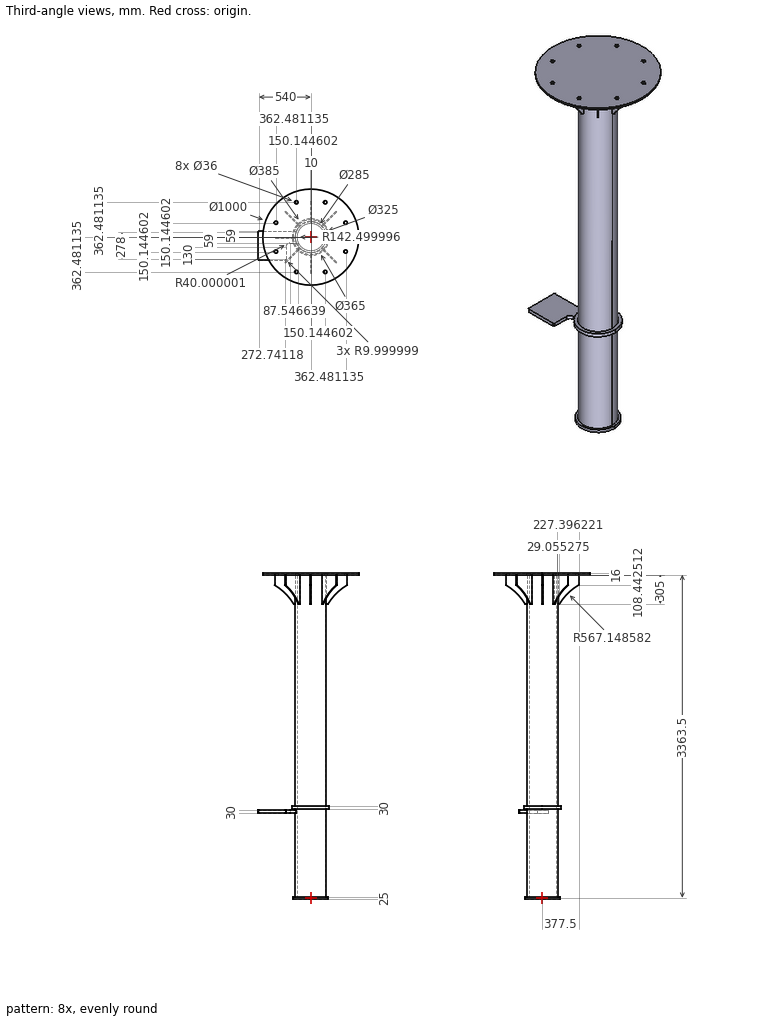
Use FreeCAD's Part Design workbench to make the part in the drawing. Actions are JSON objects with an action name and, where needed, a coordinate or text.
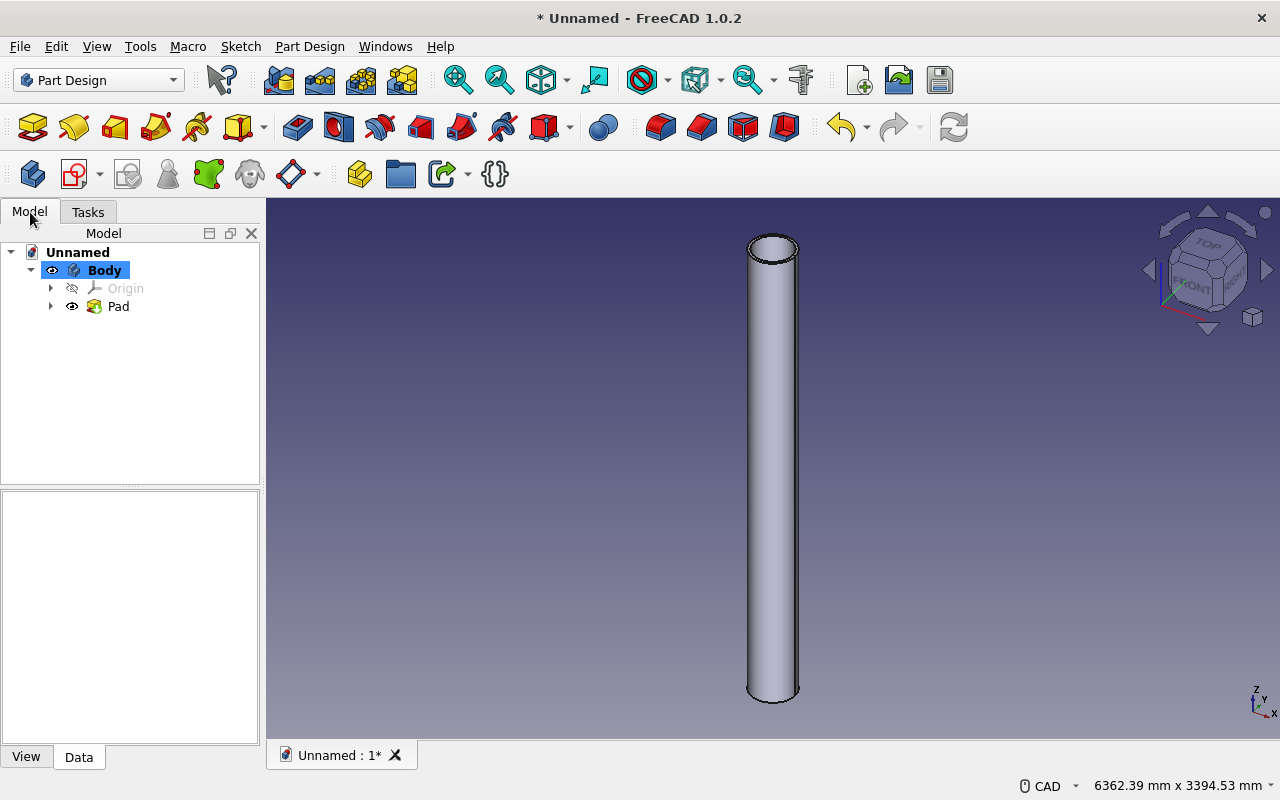
{"action": "left_click", "coordinate": [51, 288]}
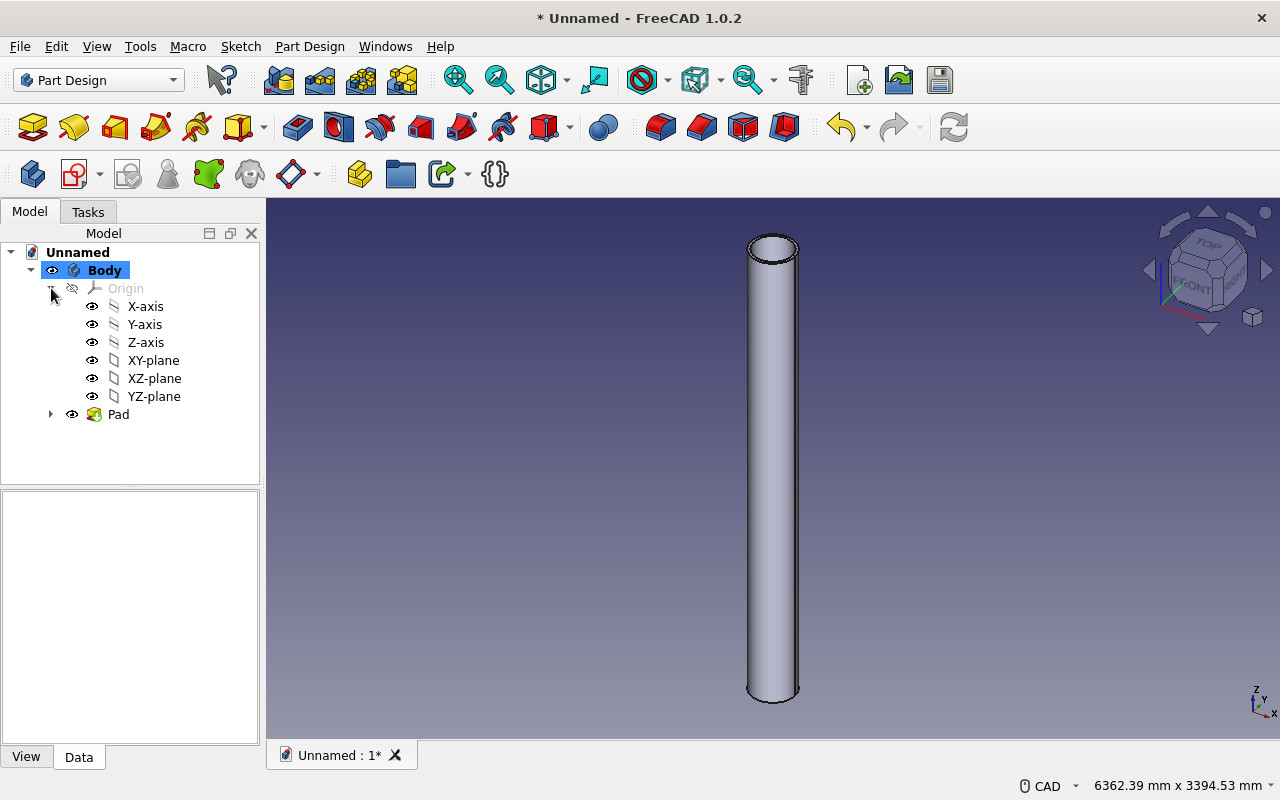
{"action": "left_click", "coordinate": [137, 360]}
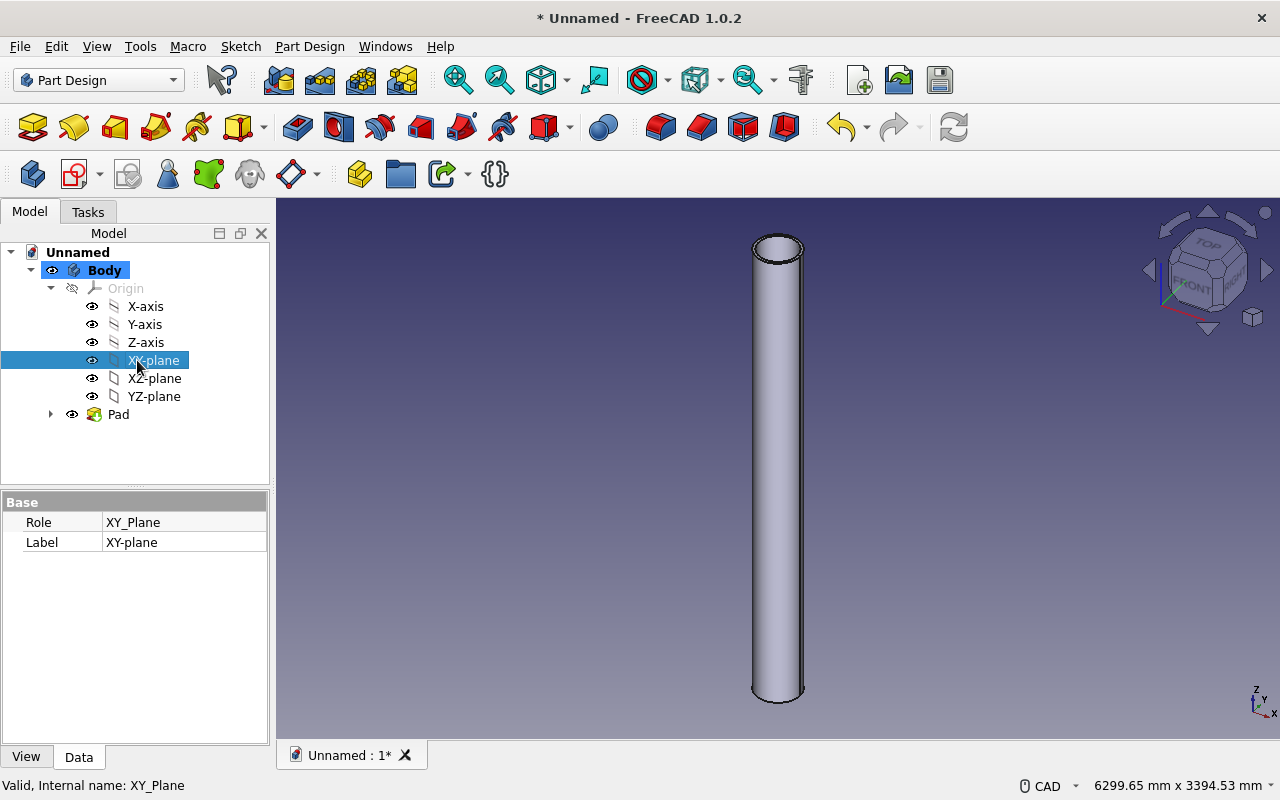
{"action": "left_click", "coordinate": [290, 174]}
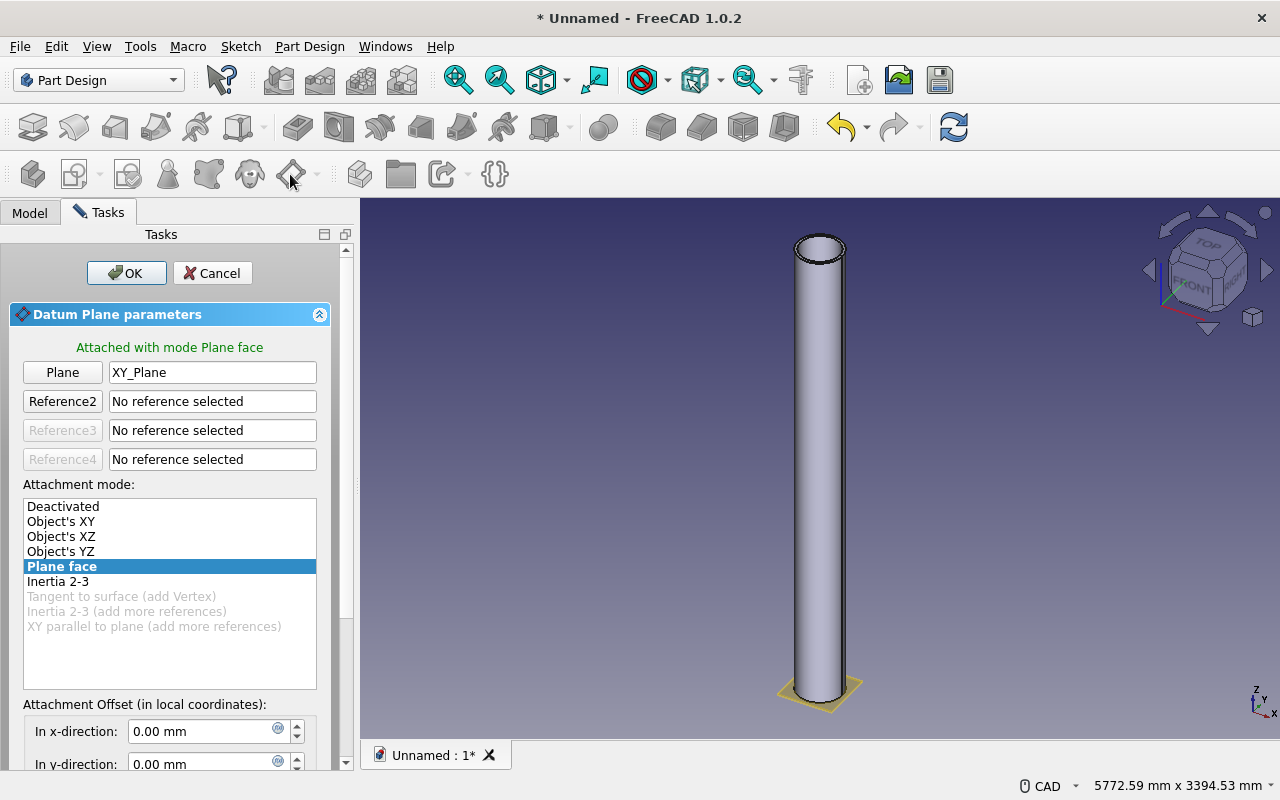
{"action": "scroll", "coordinate": [346, 507], "scroll_direction": "down", "scroll_amount": 2}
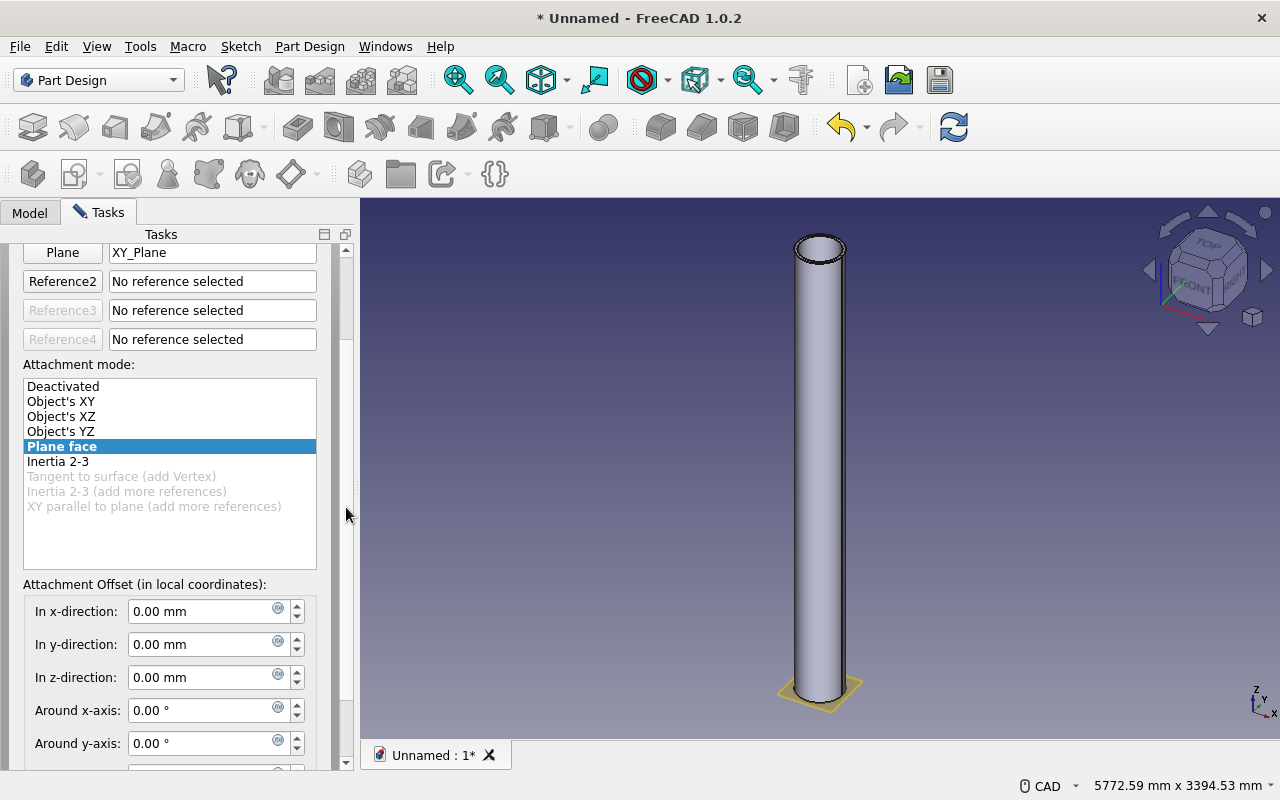
{"action": "triple_click", "coordinate": [210, 678]}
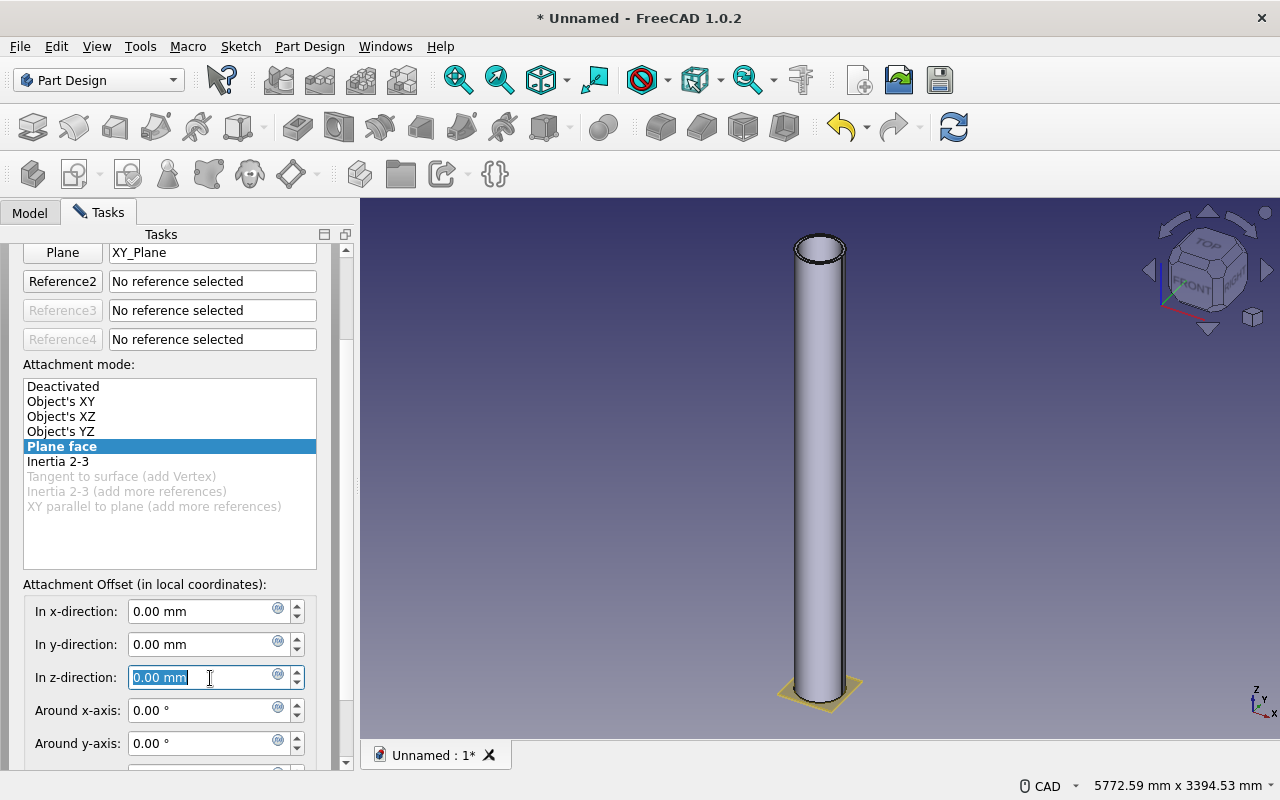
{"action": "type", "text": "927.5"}
{"action": "key", "text": "Tab"}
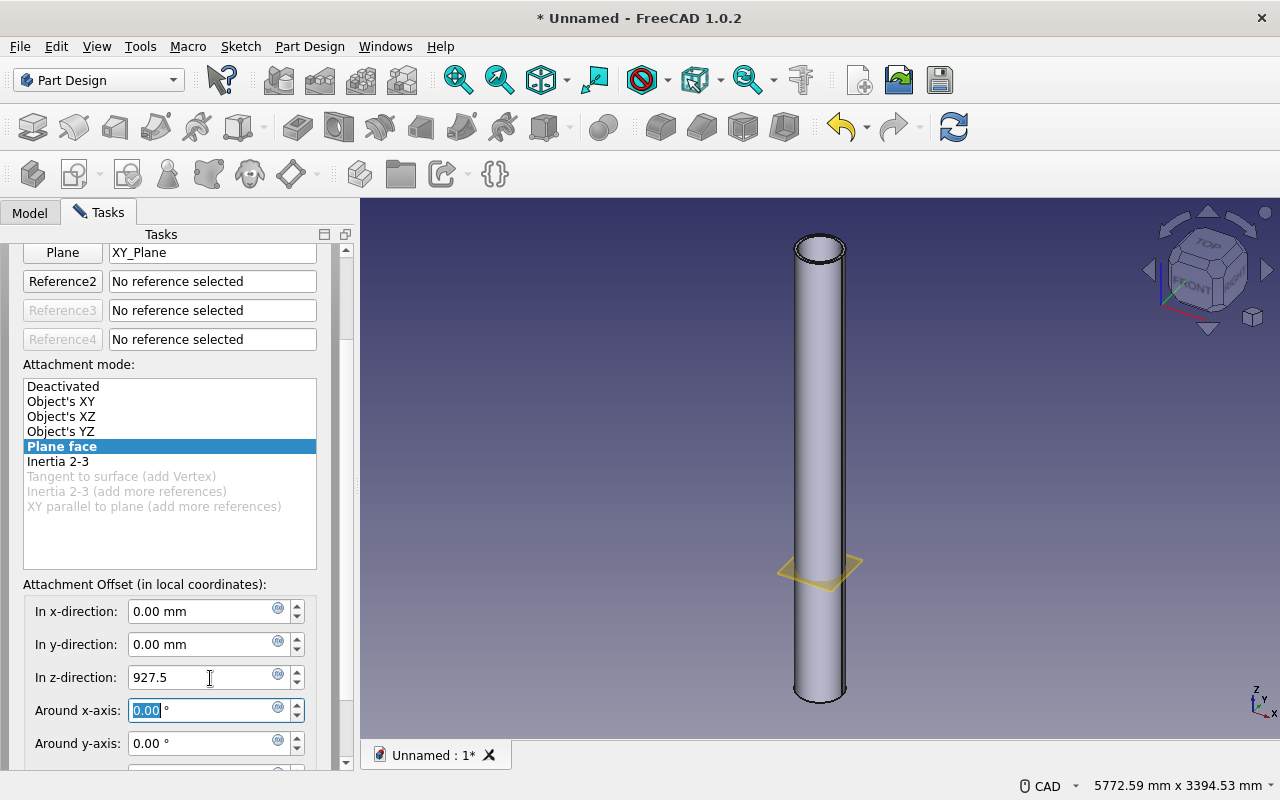
{"action": "scroll", "coordinate": [346, 507], "scroll_direction": "up", "scroll_amount": 3}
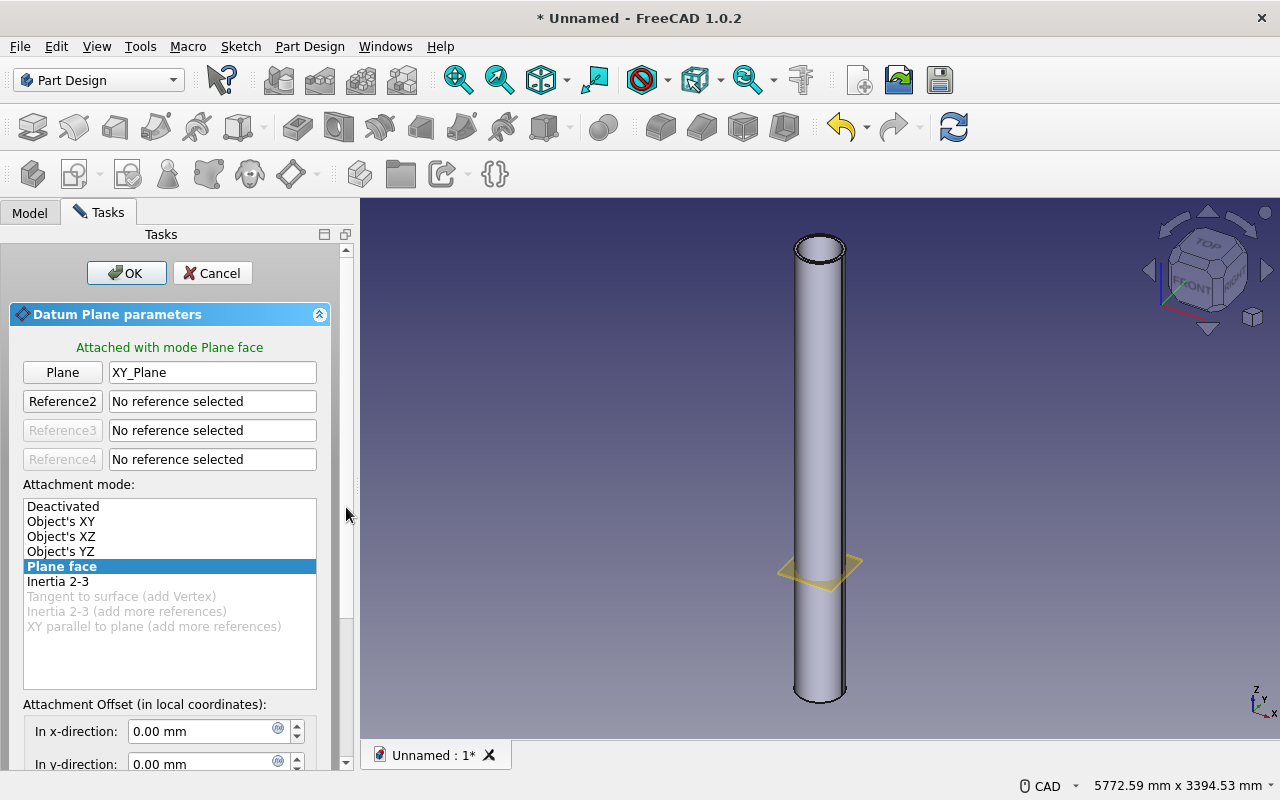
{"action": "left_click", "coordinate": [127, 273]}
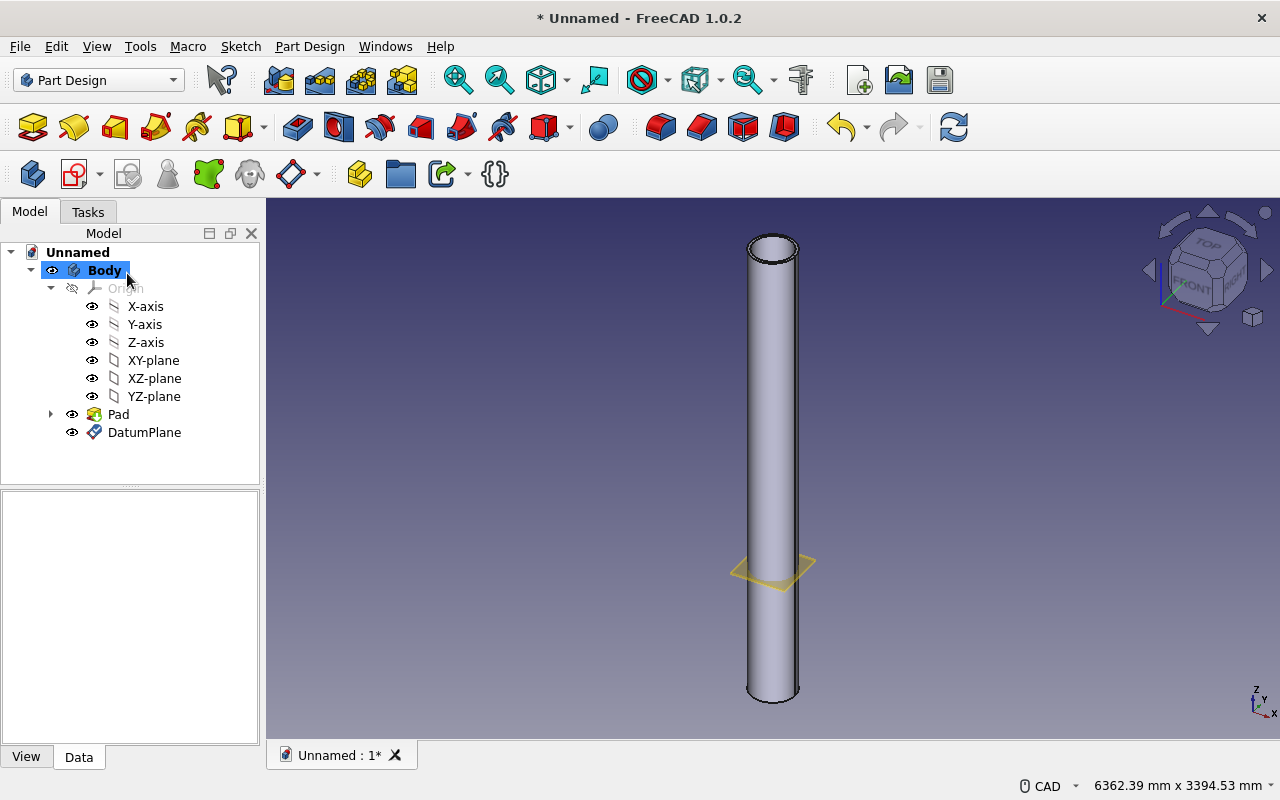
{"action": "left_click", "coordinate": [117, 432]}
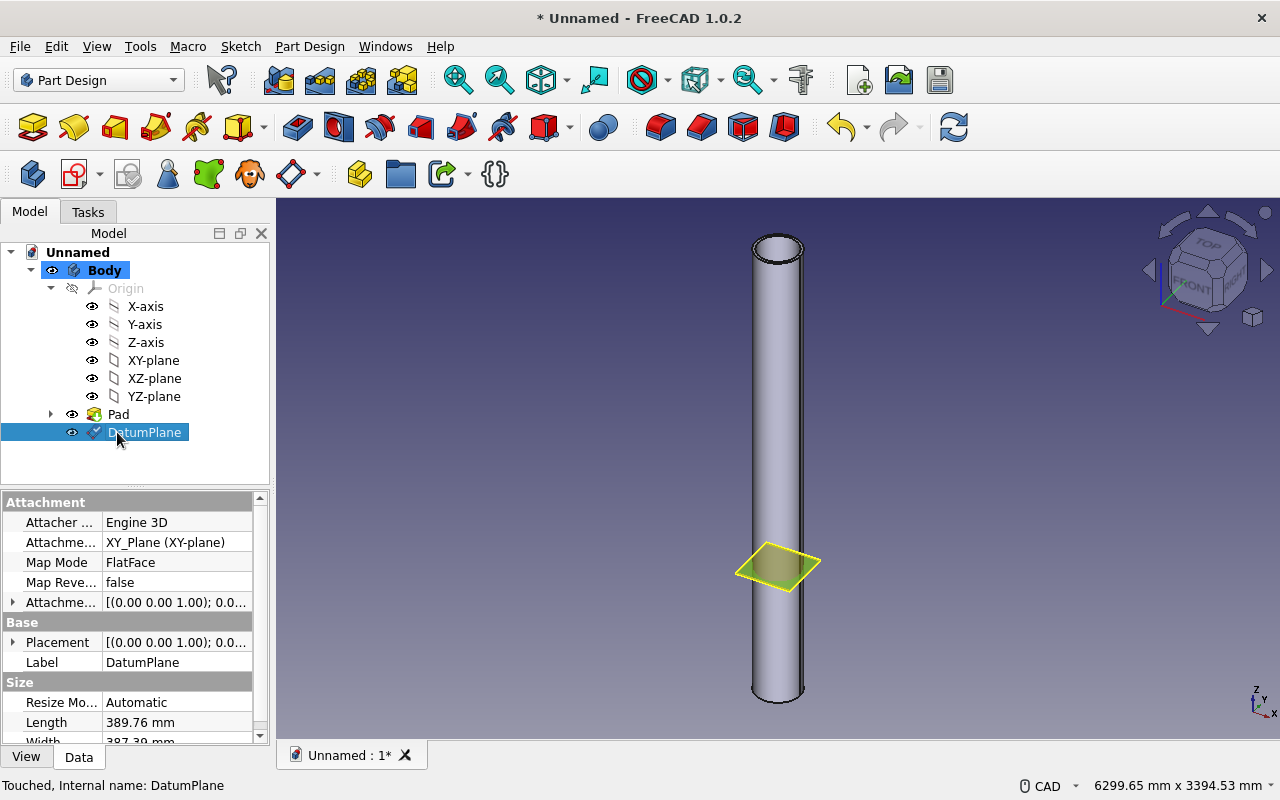
{"action": "left_click", "coordinate": [74, 174]}